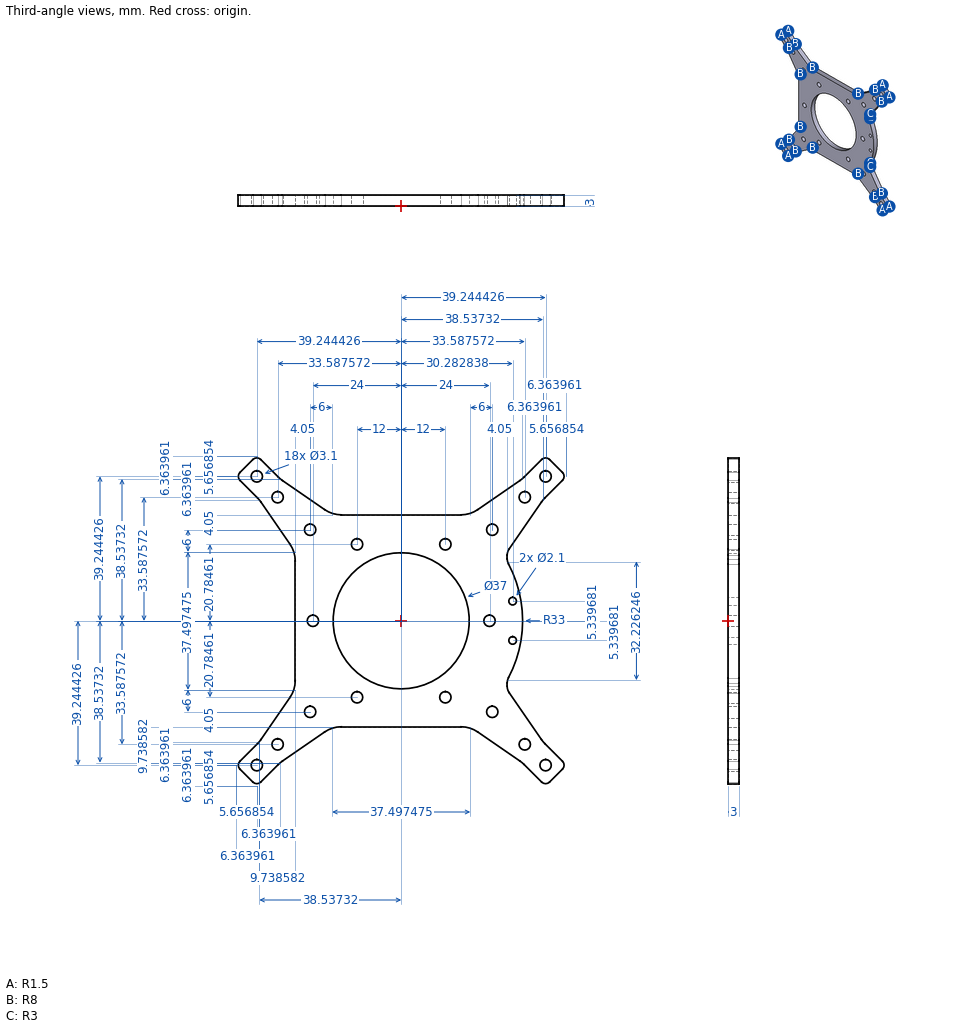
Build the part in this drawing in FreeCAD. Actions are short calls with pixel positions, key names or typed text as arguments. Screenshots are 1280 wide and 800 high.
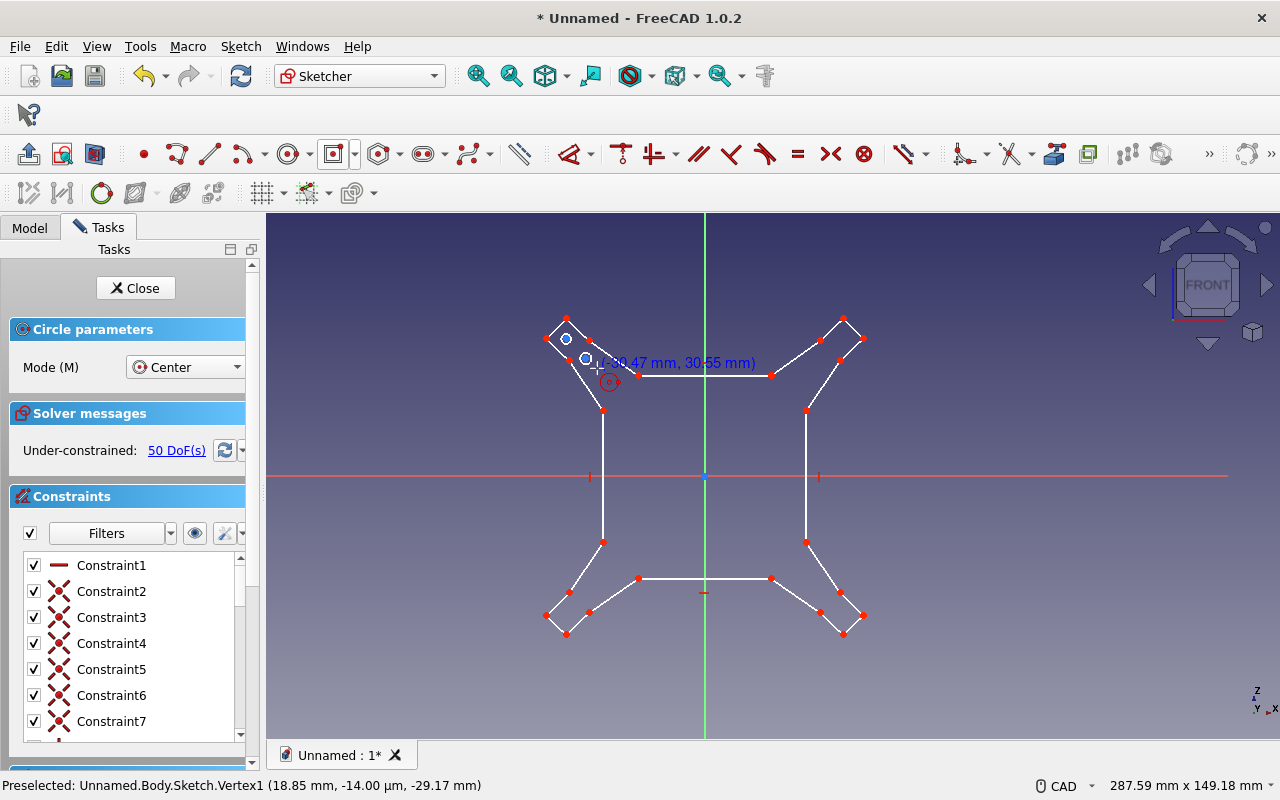
click(617, 389)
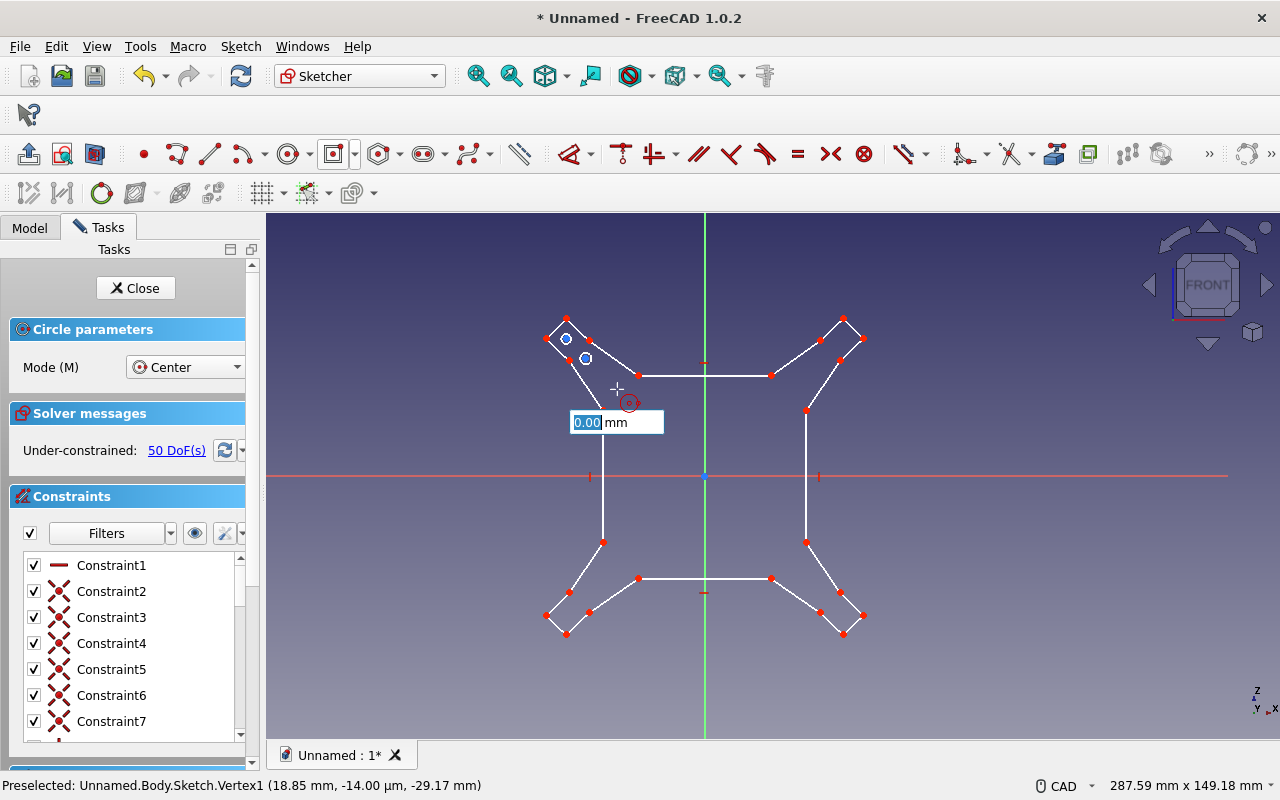
scroll(621, 385, up, 6)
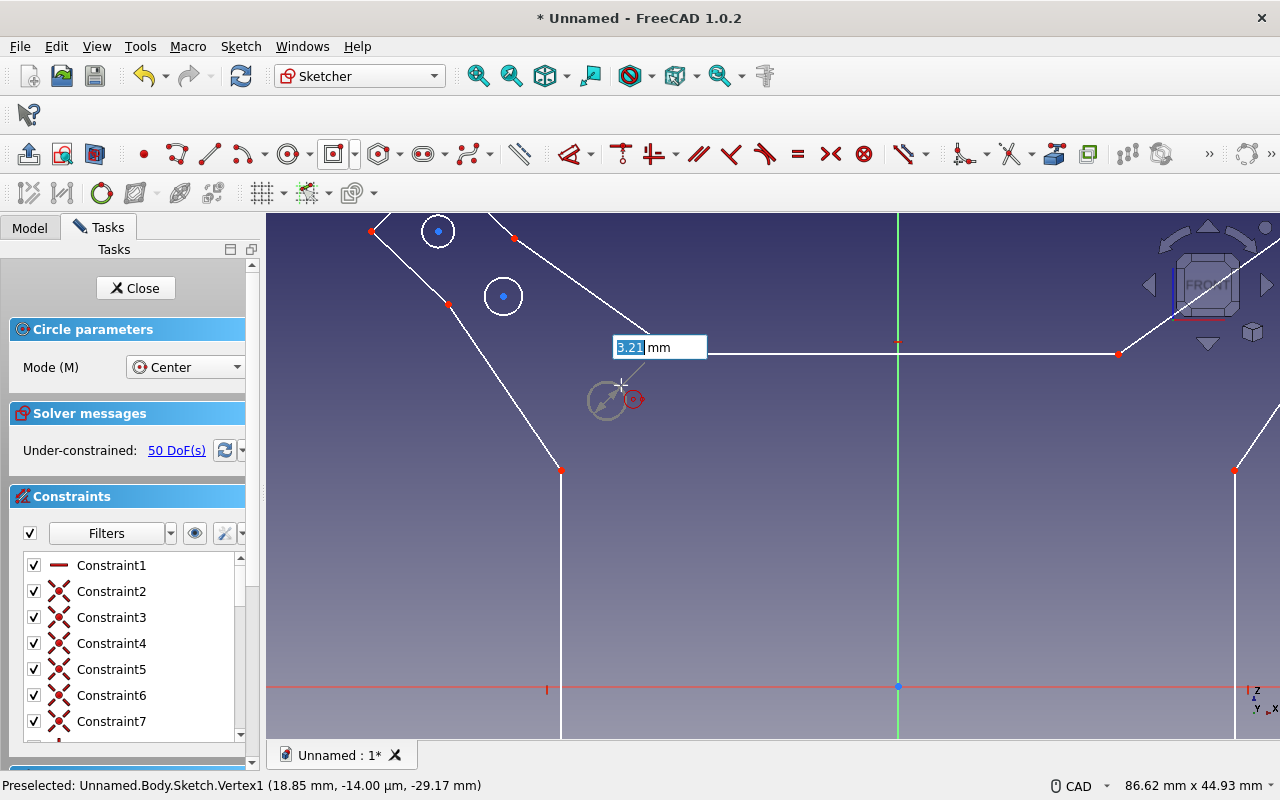
click(621, 384)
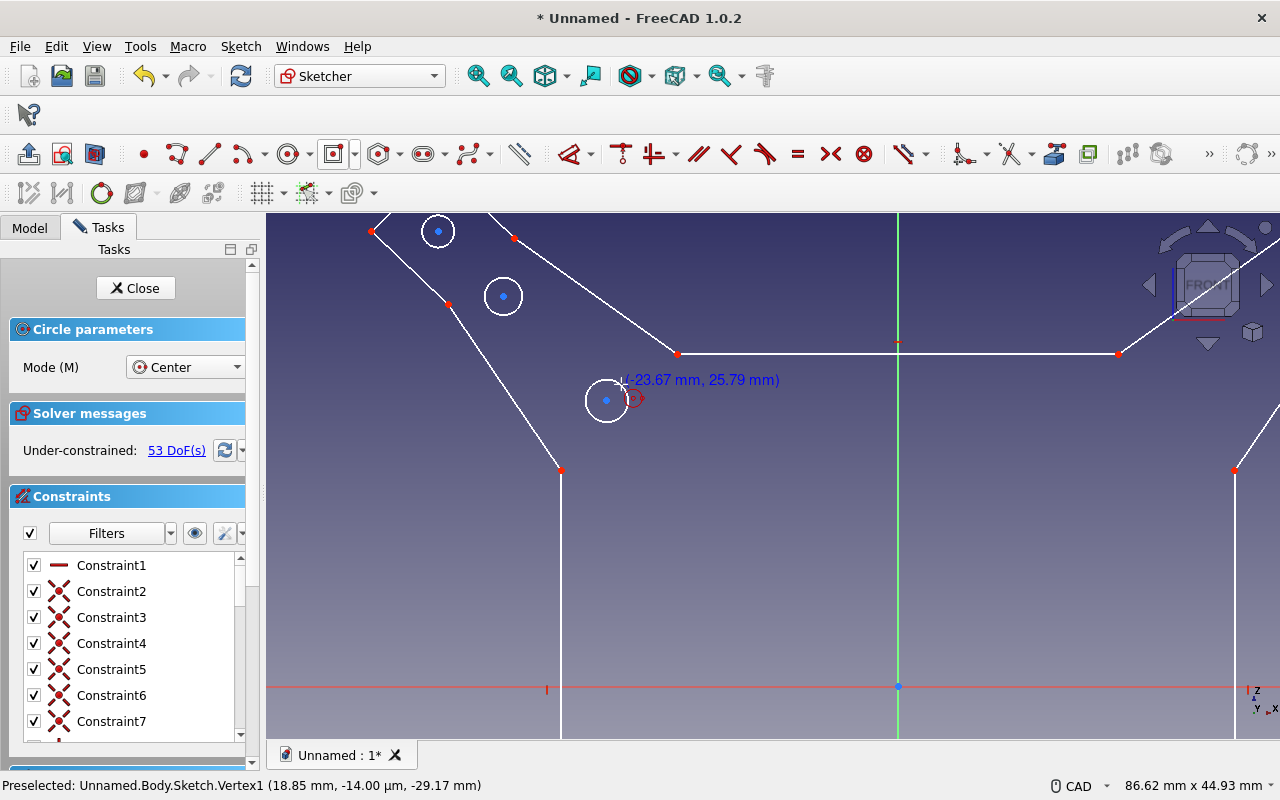
scroll(758, 444, up, 2)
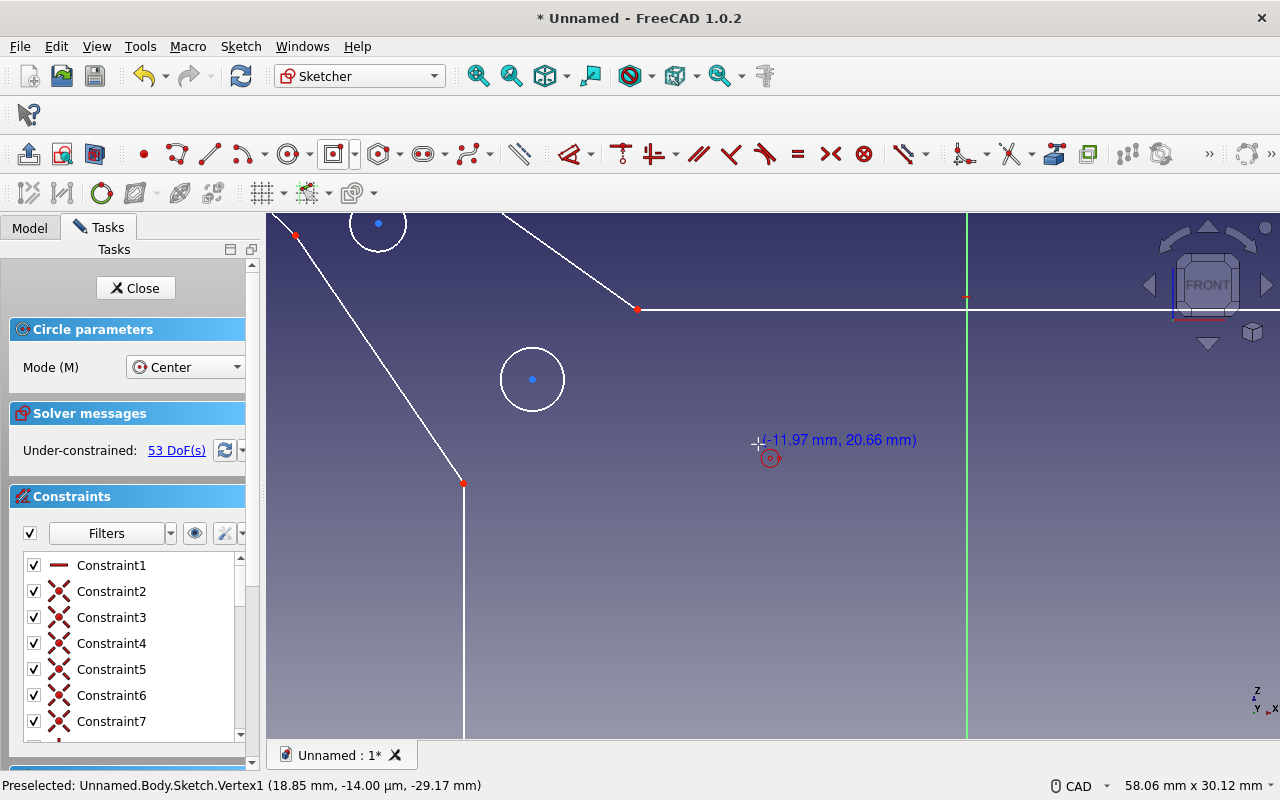
scroll(638, 393, down, 8)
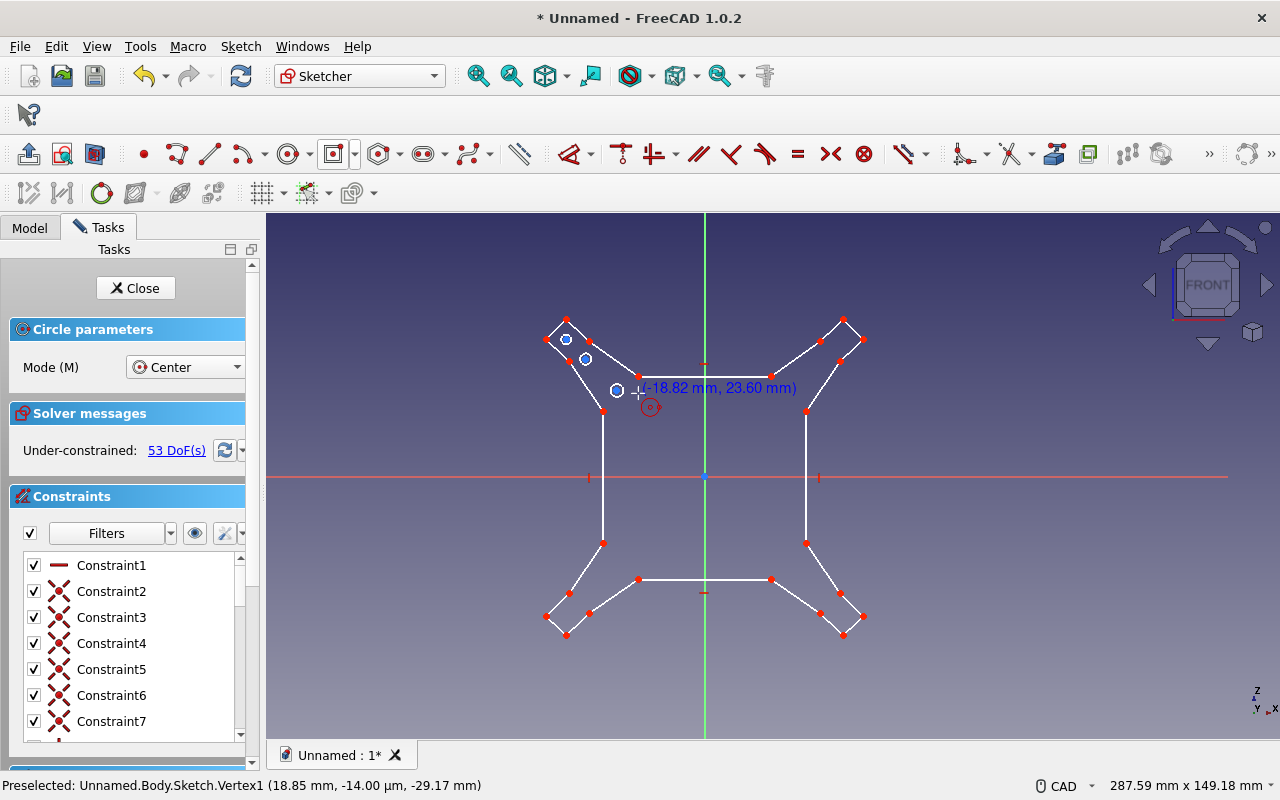
click(662, 403)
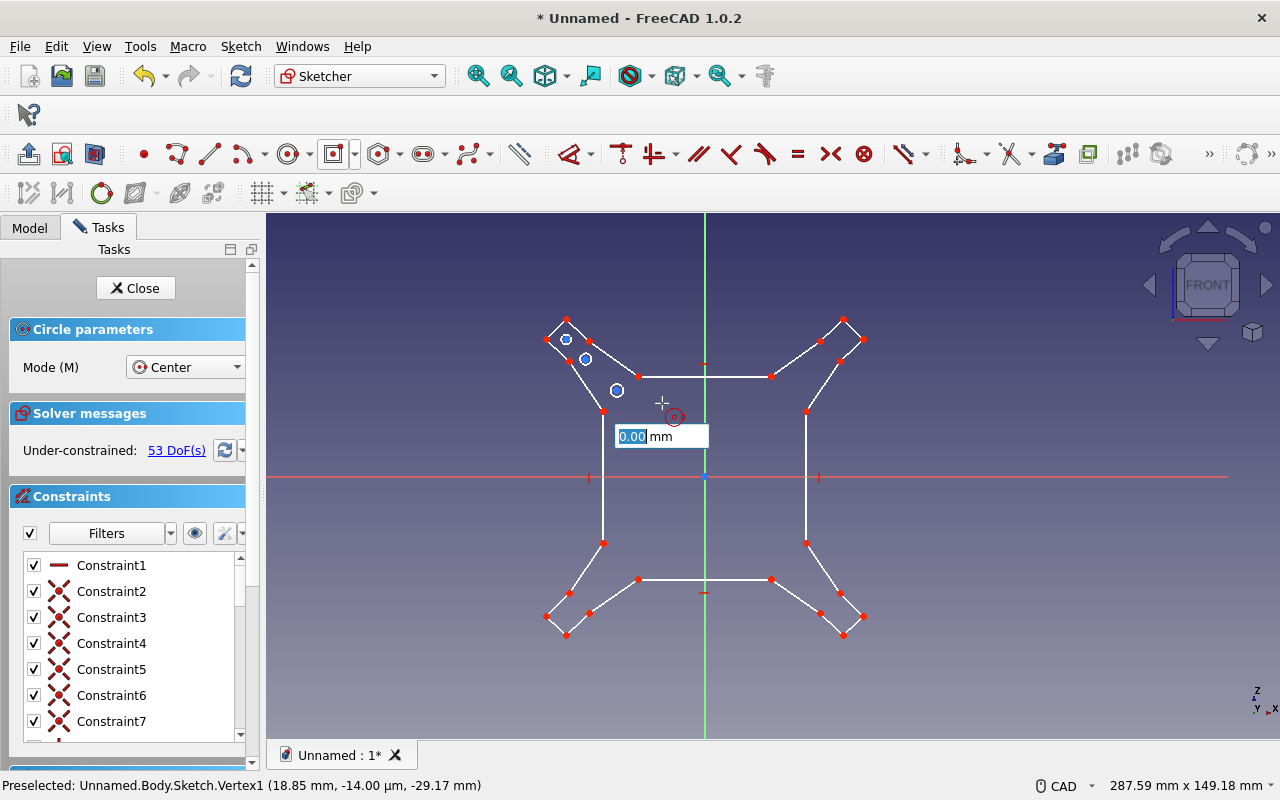
scroll(666, 400, up, 6)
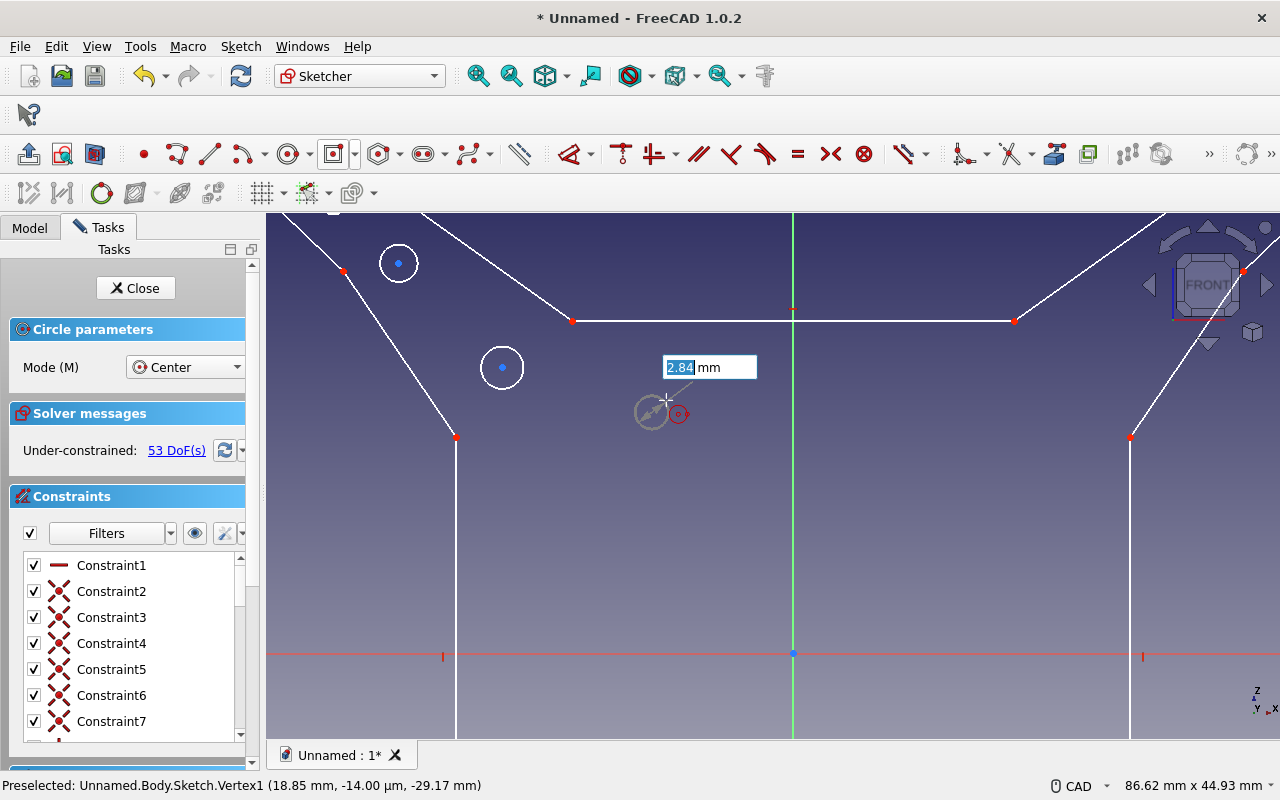
click(666, 398)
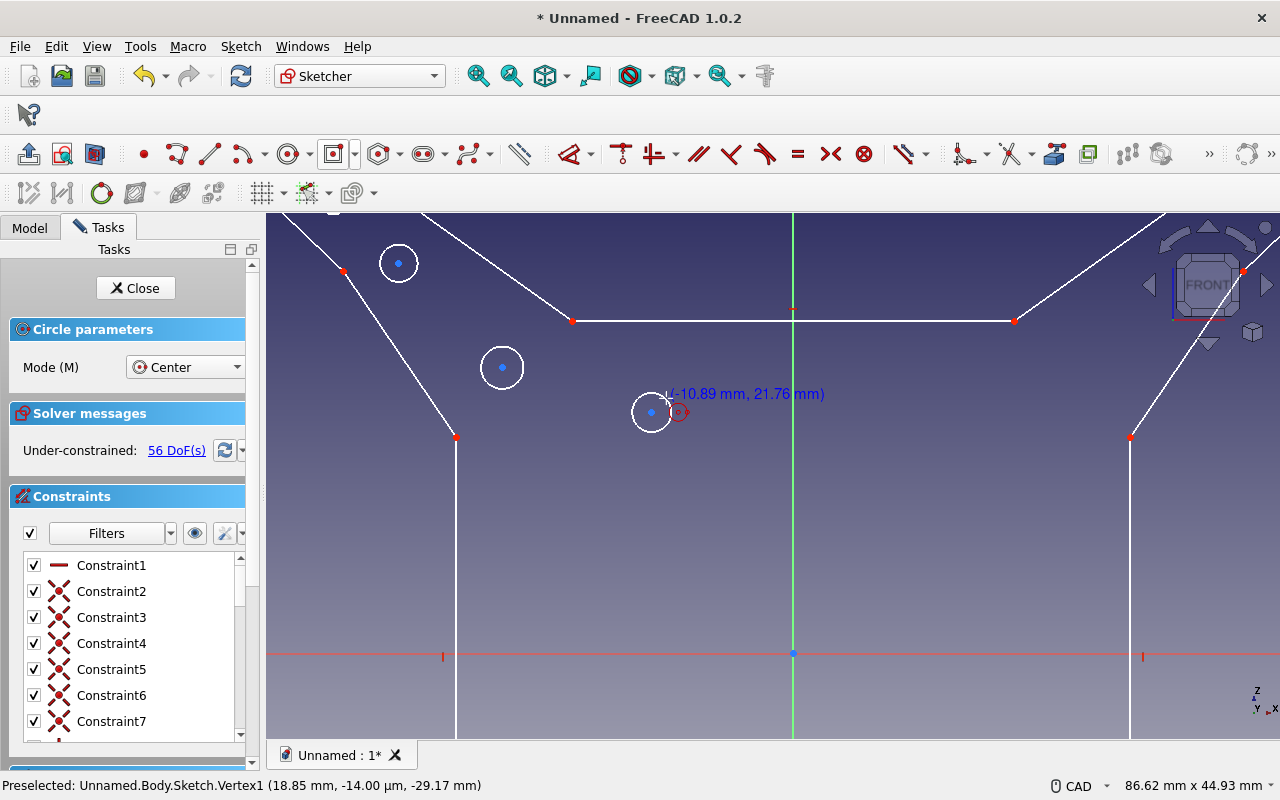
scroll(934, 410, up, 2)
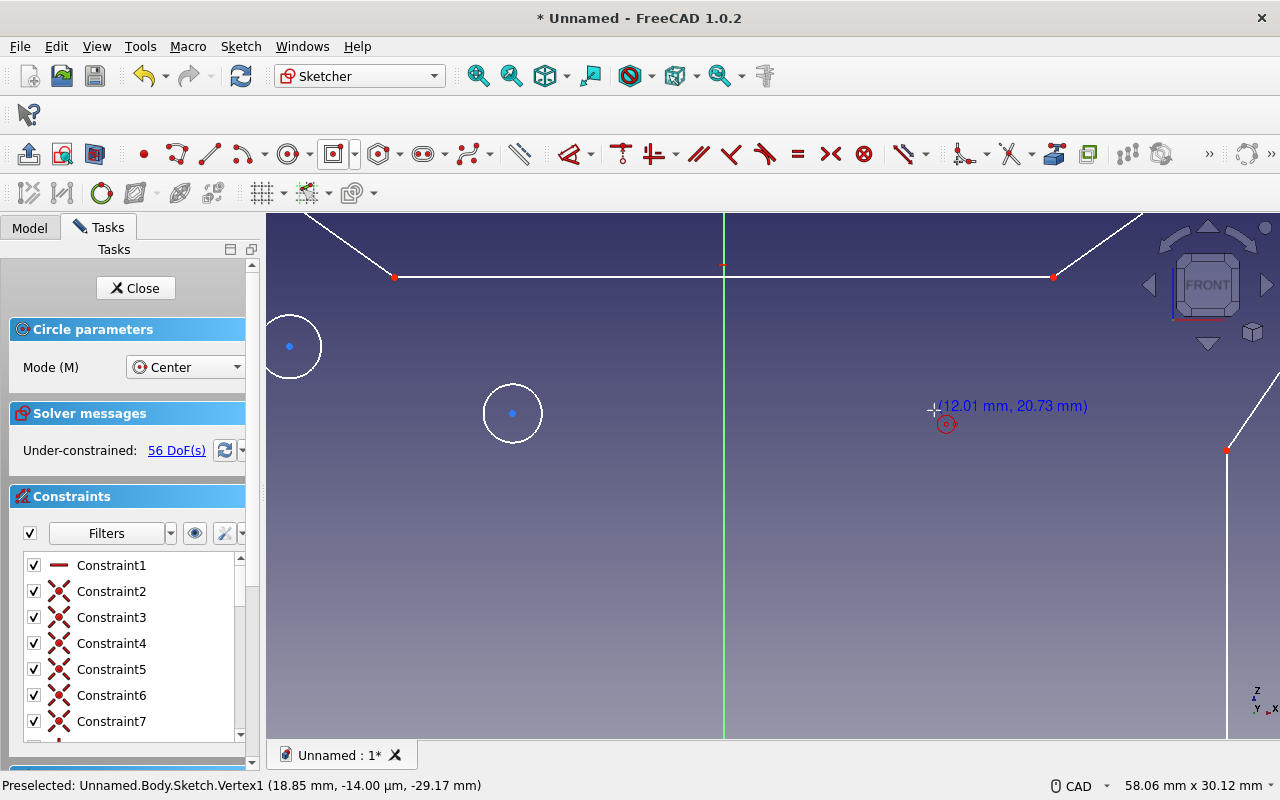
scroll(700, 401, down, 8)